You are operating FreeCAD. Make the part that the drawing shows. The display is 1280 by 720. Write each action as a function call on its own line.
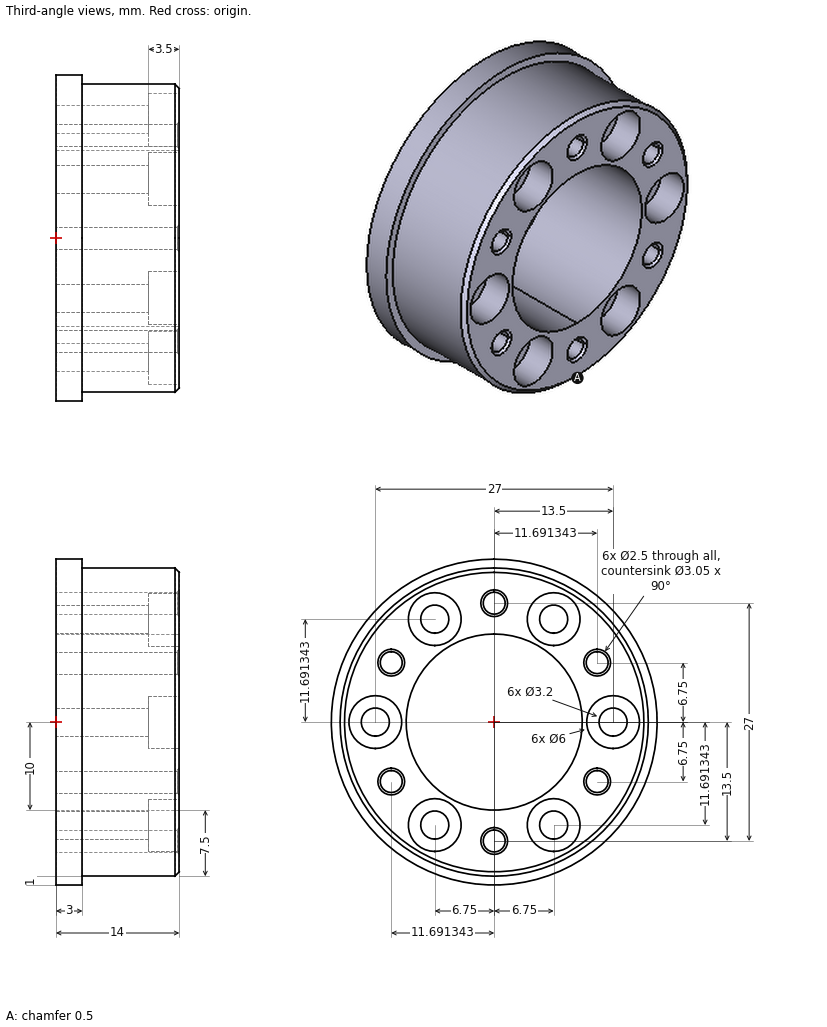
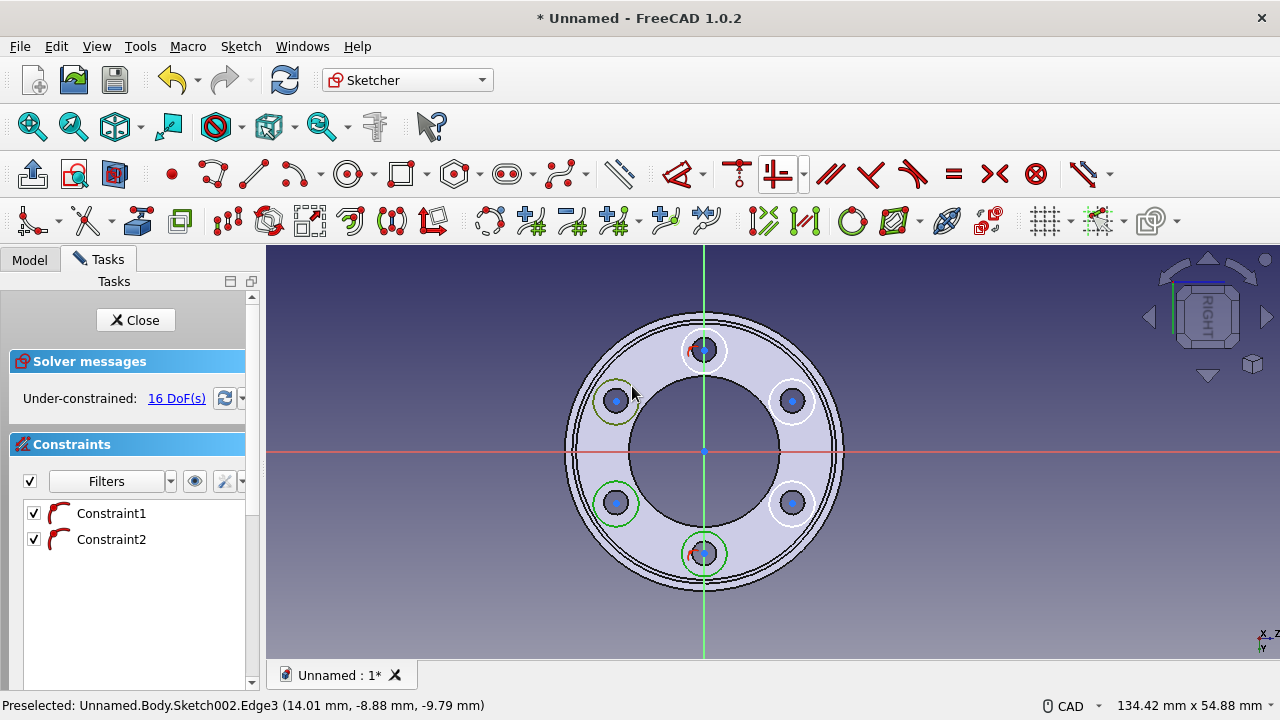
click(720, 335)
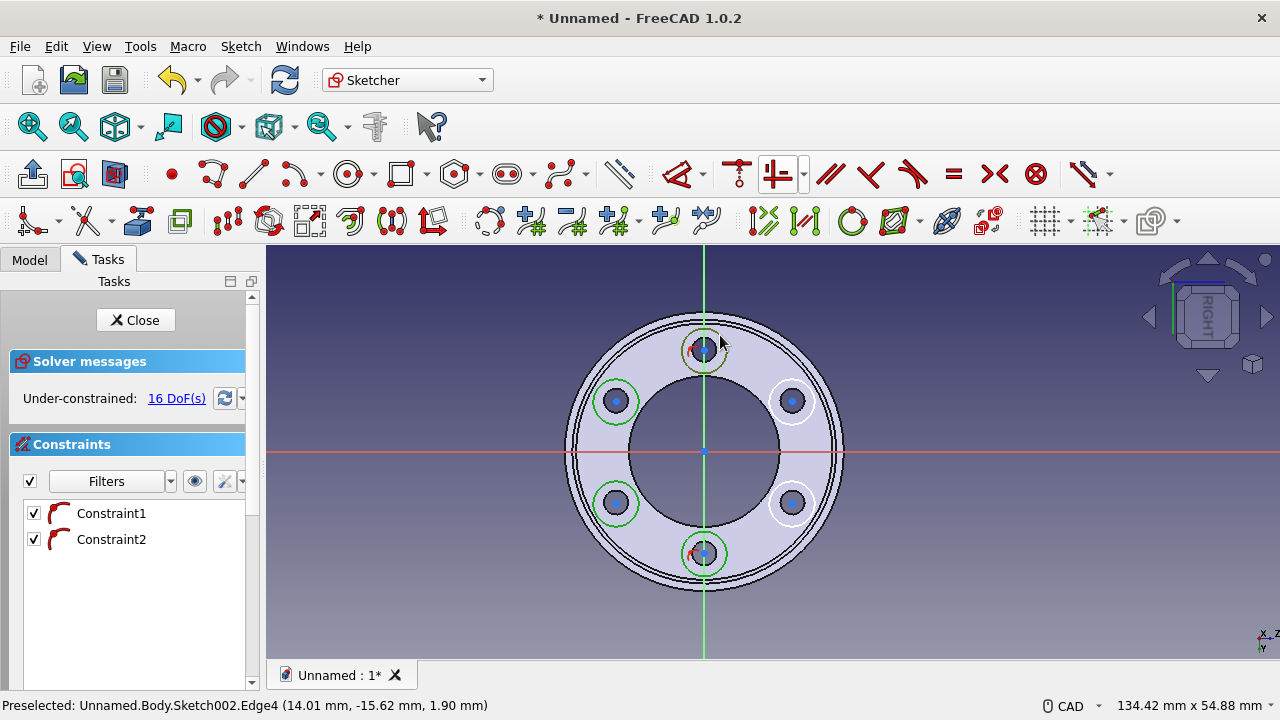
click(808, 386)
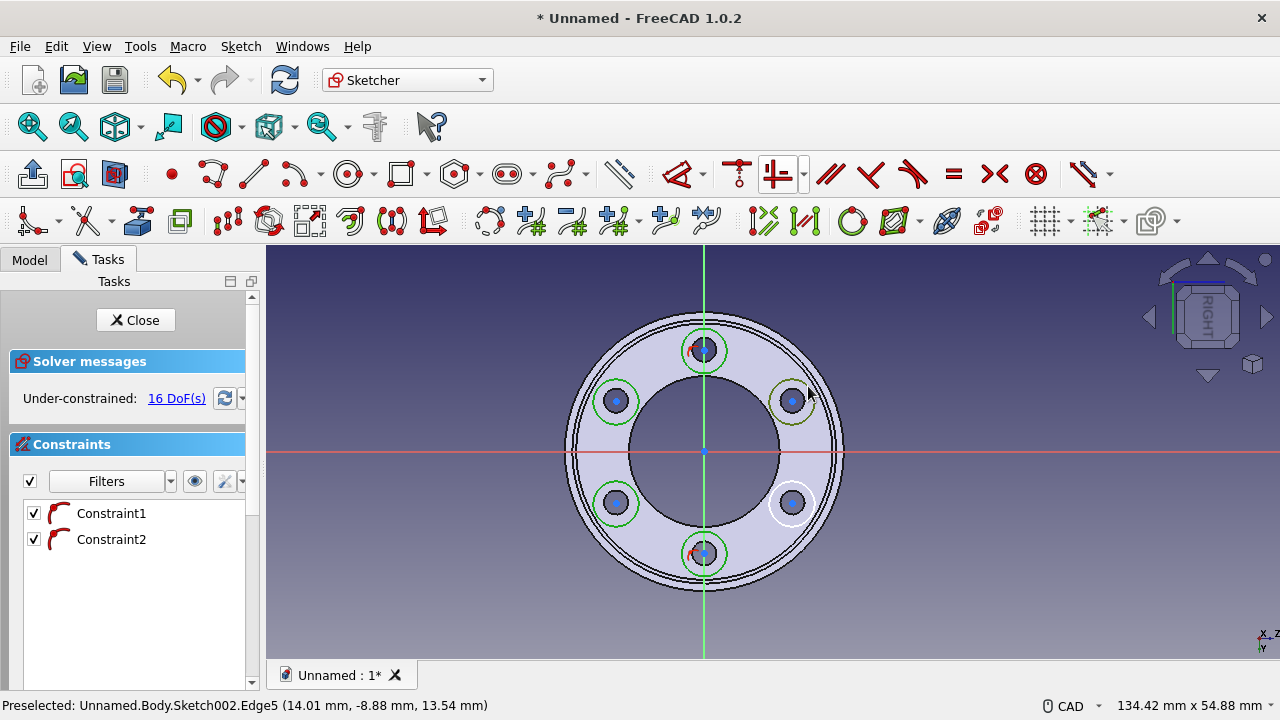
click(808, 488)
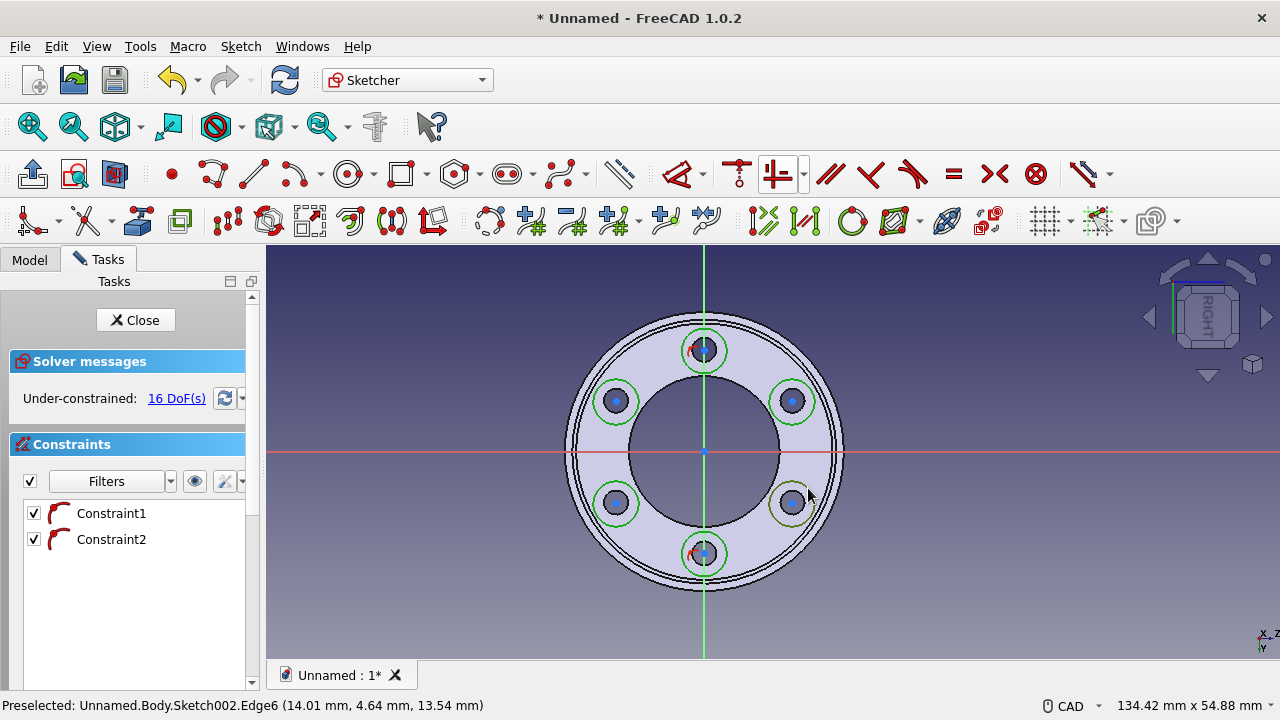
click(954, 174)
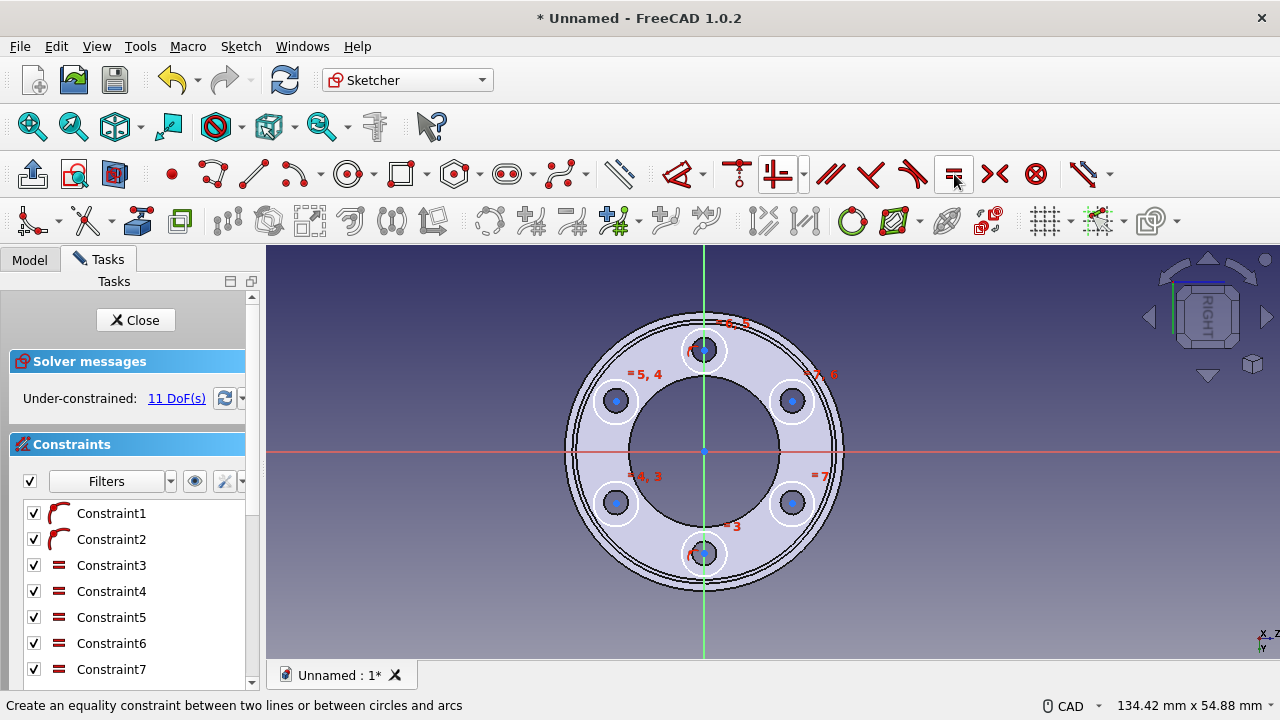
click(616, 504)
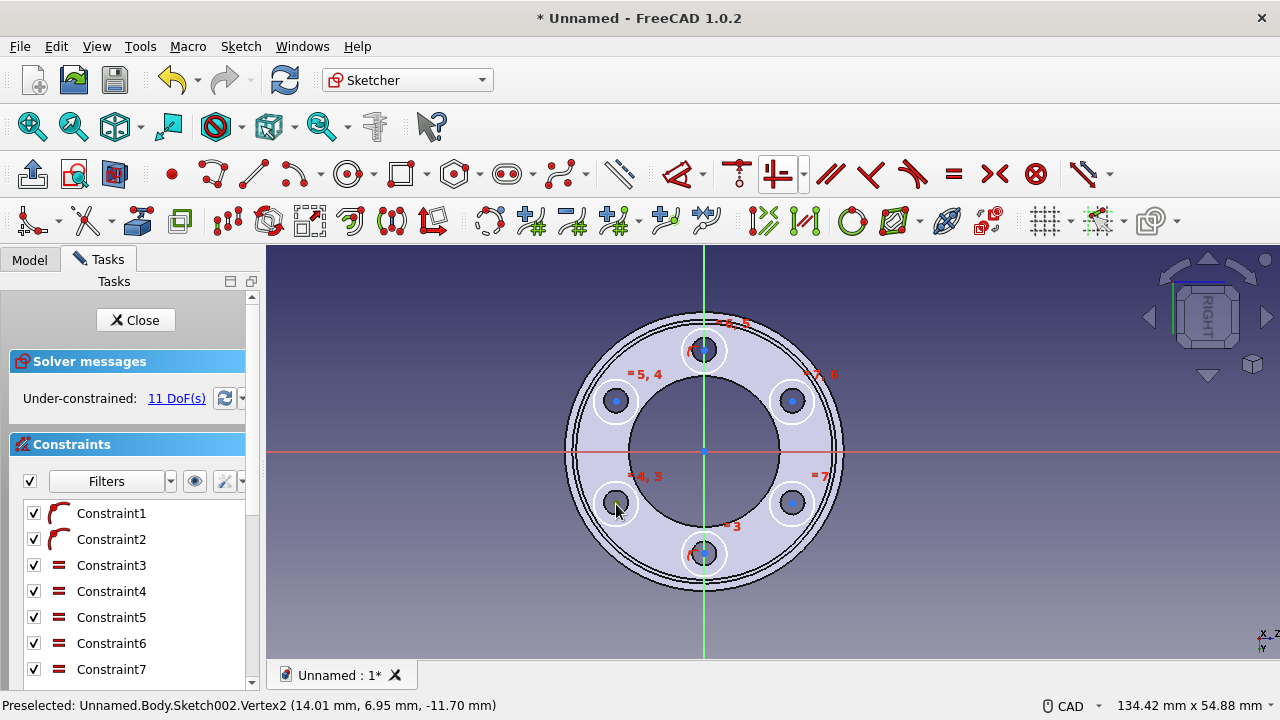
click(616, 402)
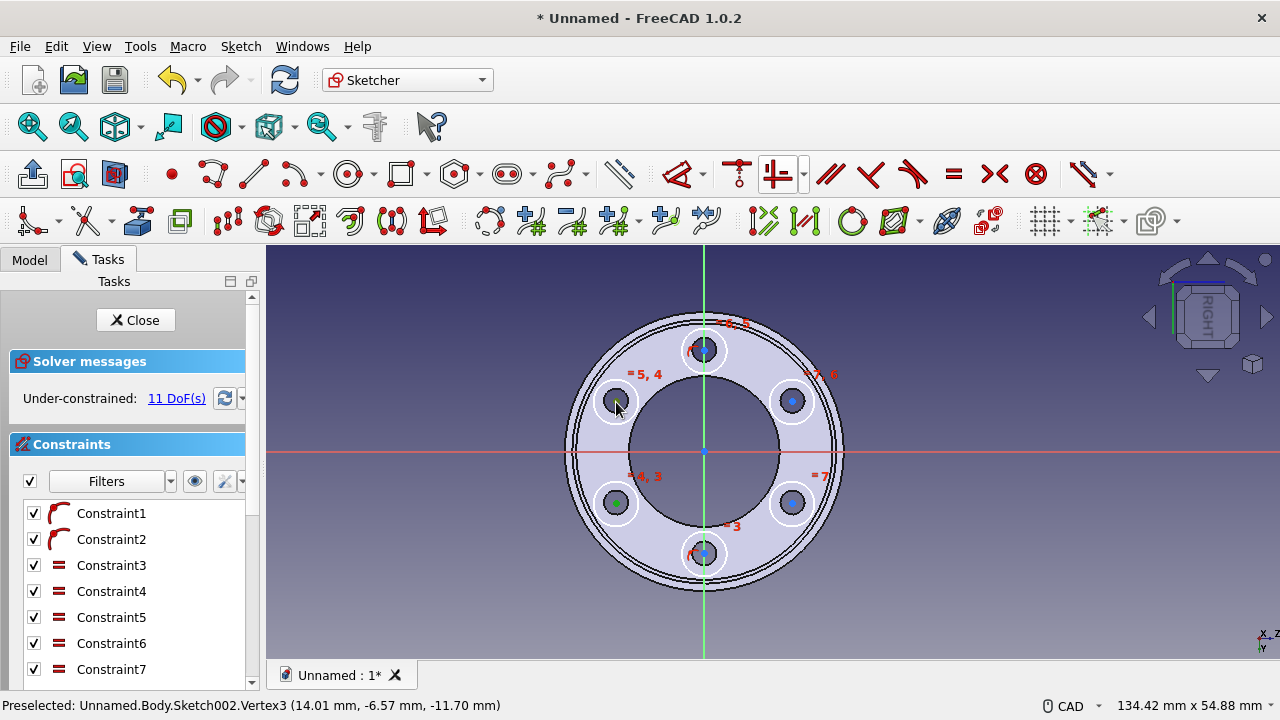
key(v)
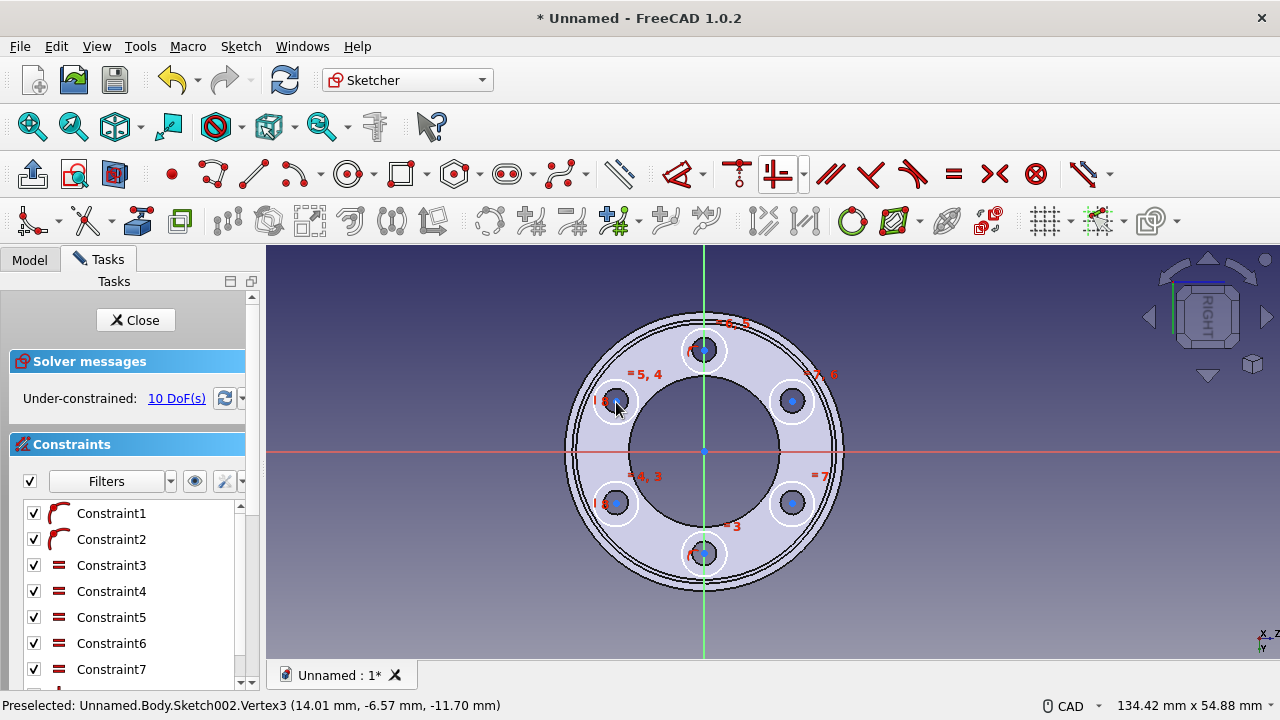
click(616, 402)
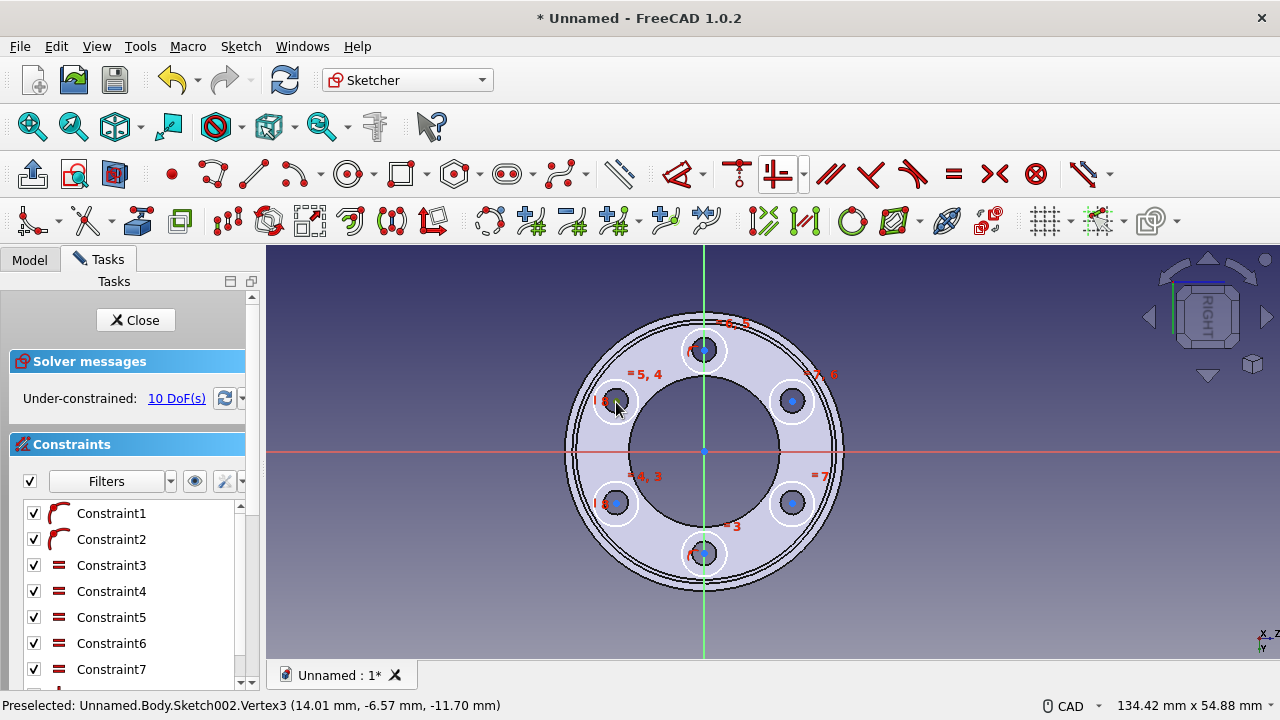
click(792, 402)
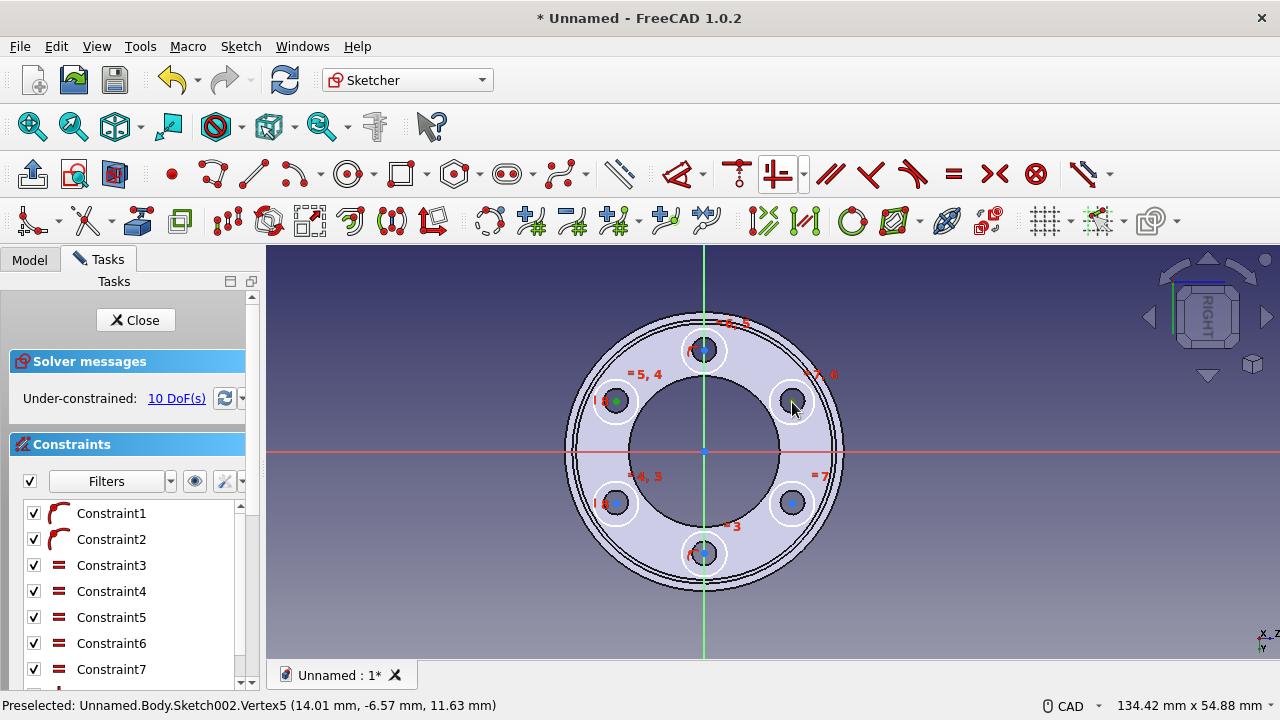
click(804, 174)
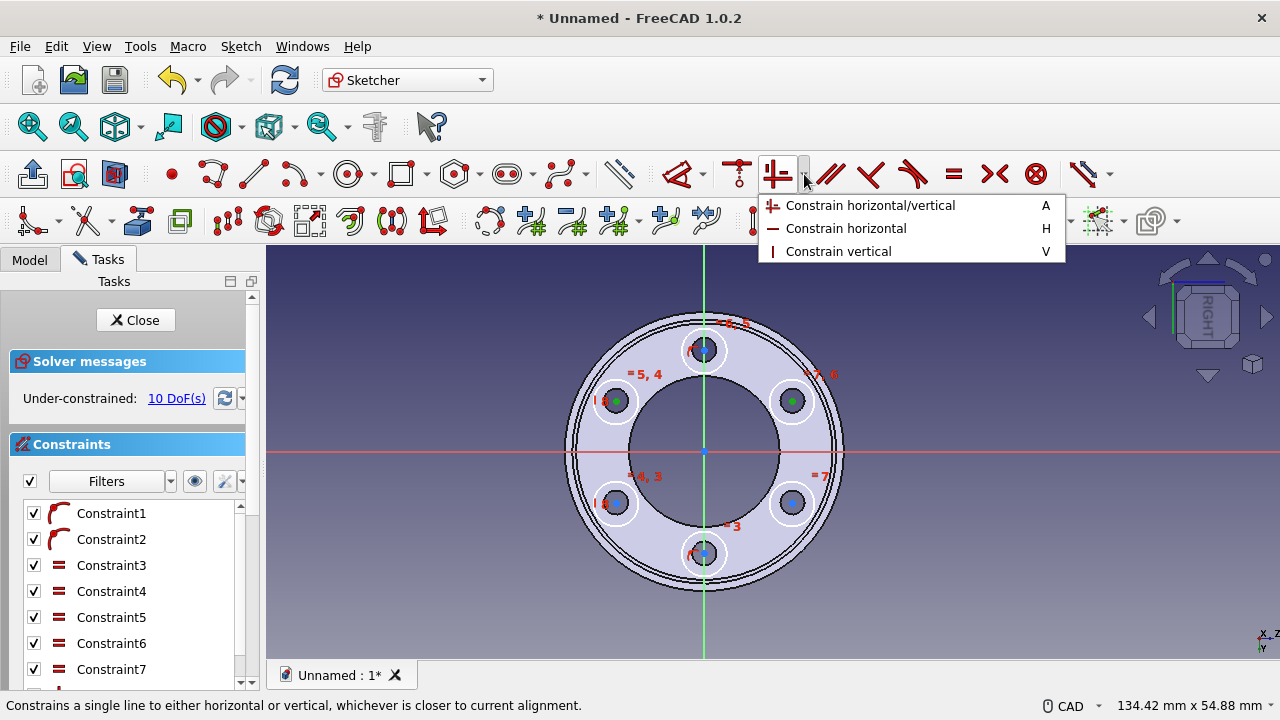
click(912, 228)